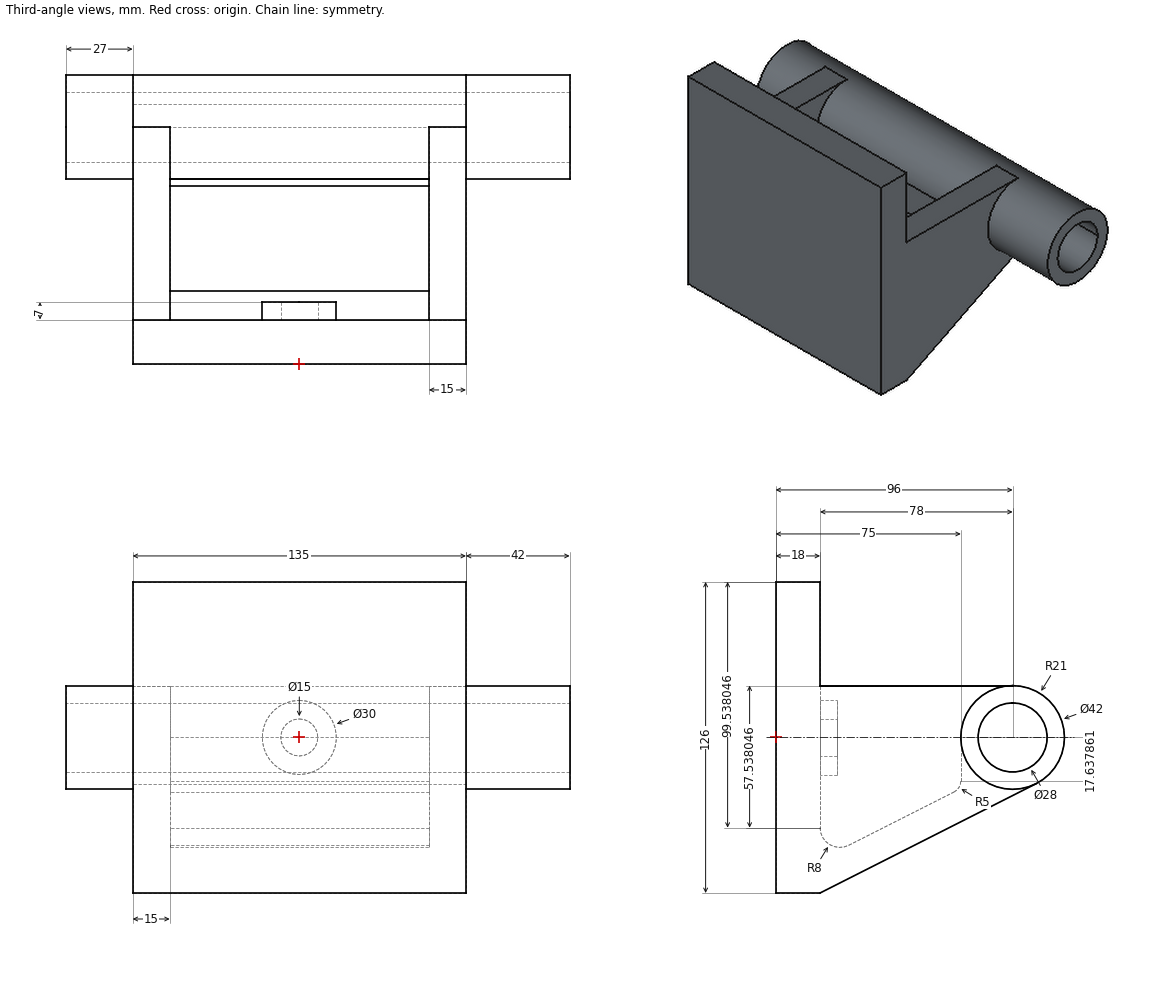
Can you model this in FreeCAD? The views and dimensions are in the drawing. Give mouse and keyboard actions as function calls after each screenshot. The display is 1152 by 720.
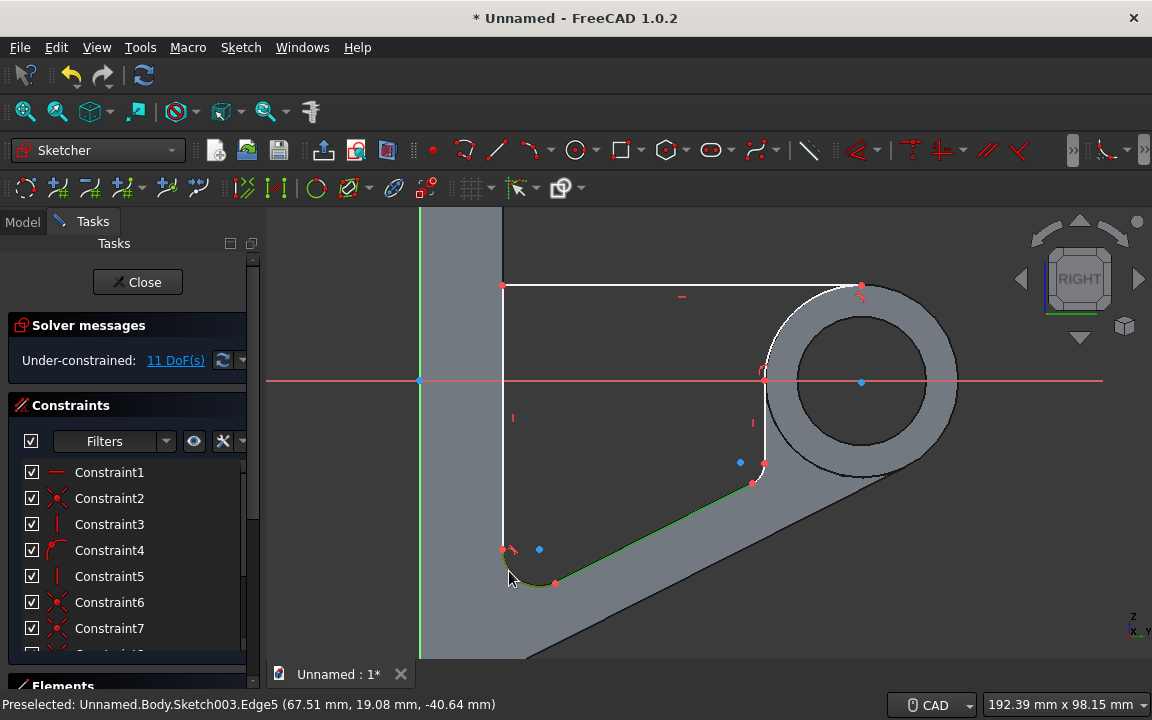
key(t)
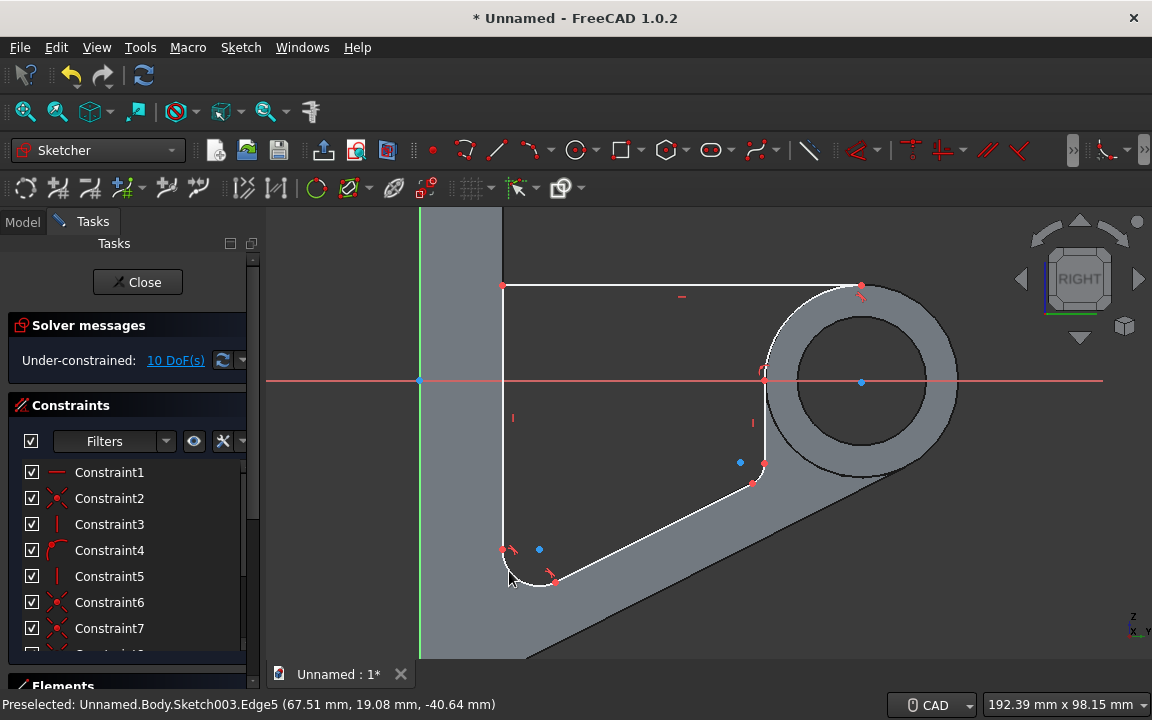
click(615, 553)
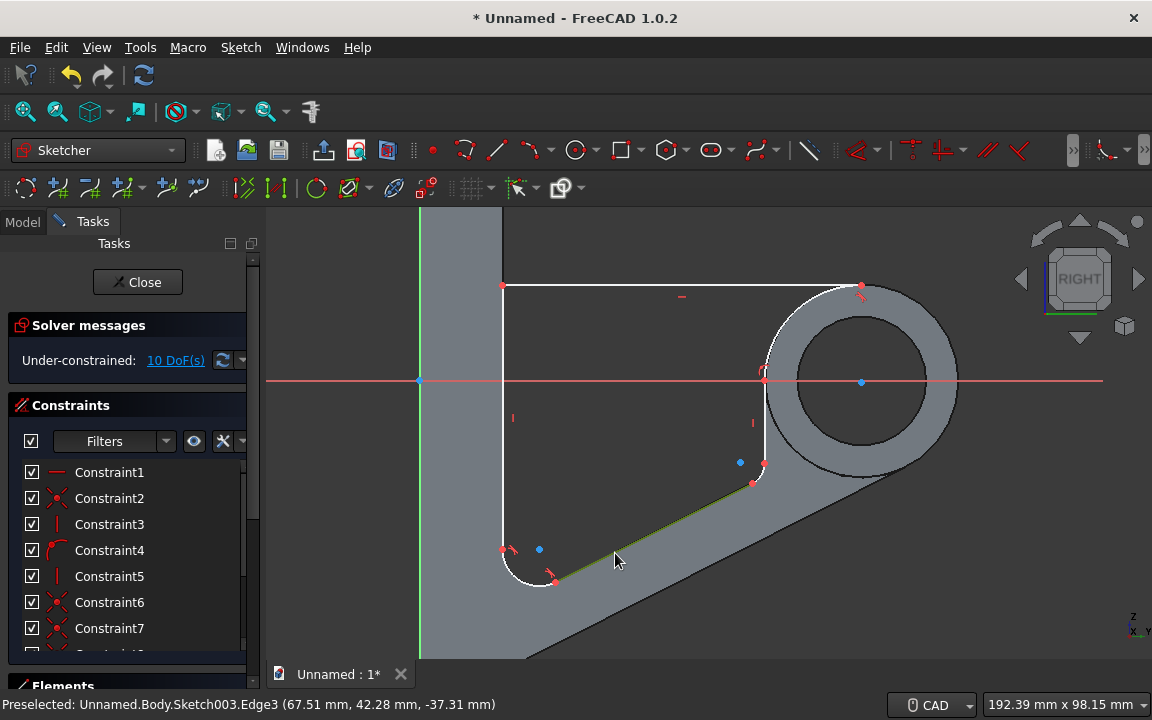
click(761, 475)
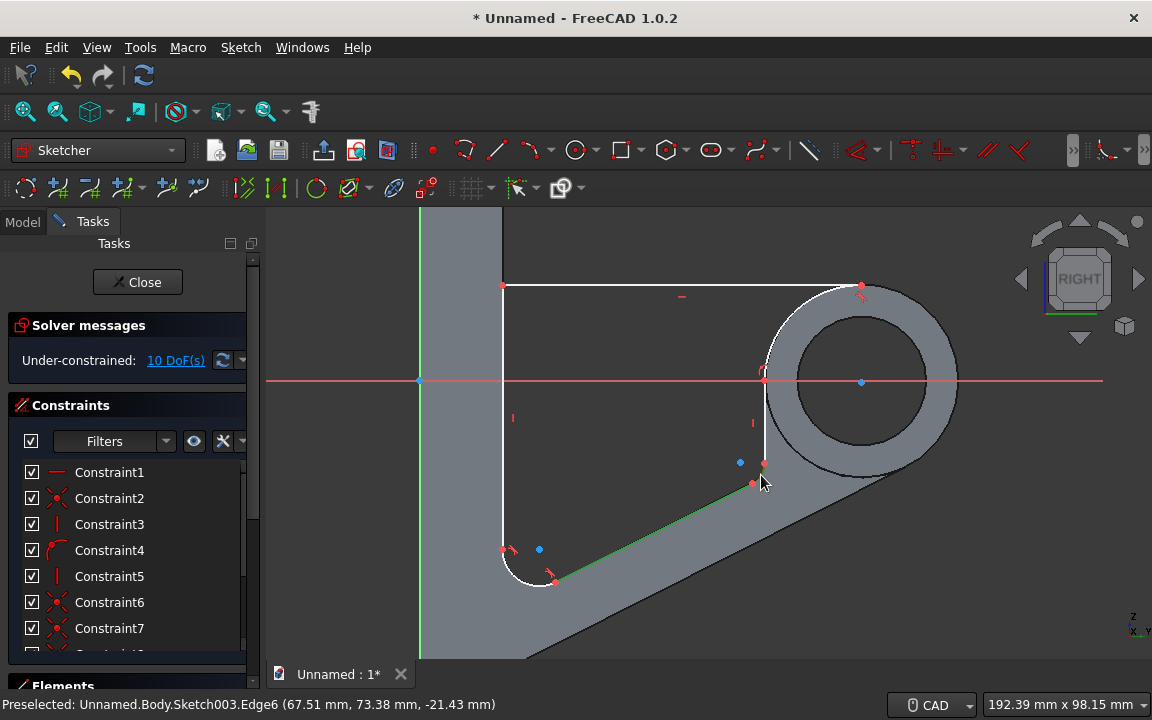
key(t)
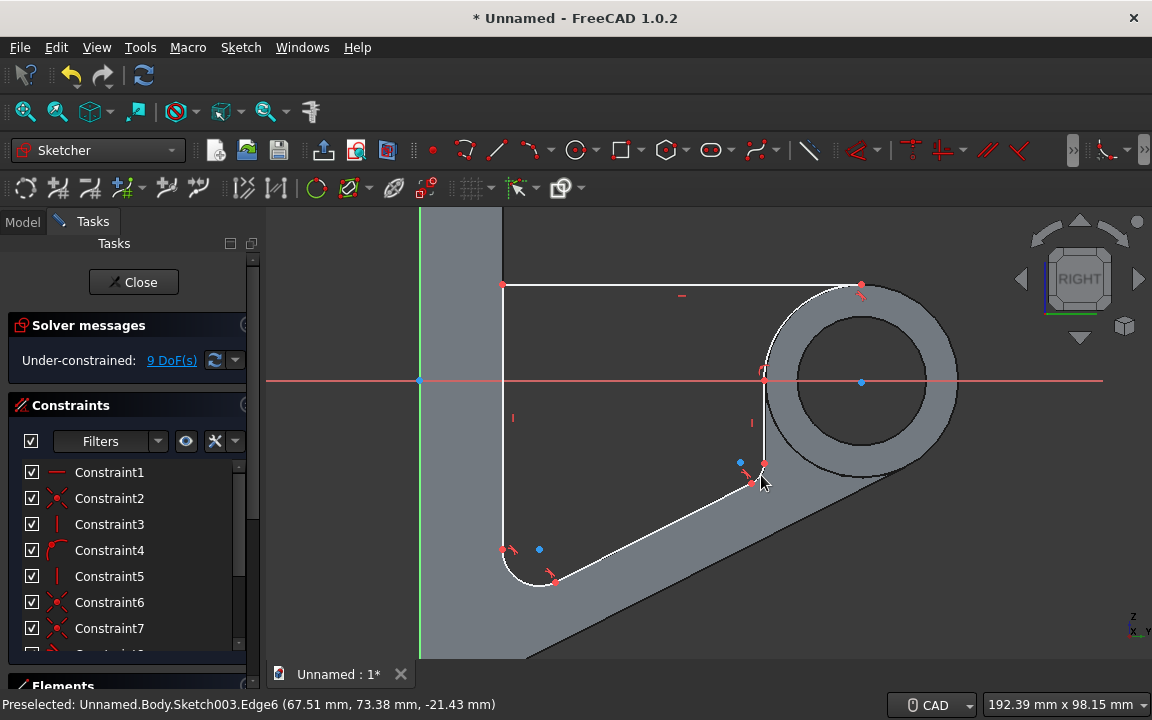
click(764, 439)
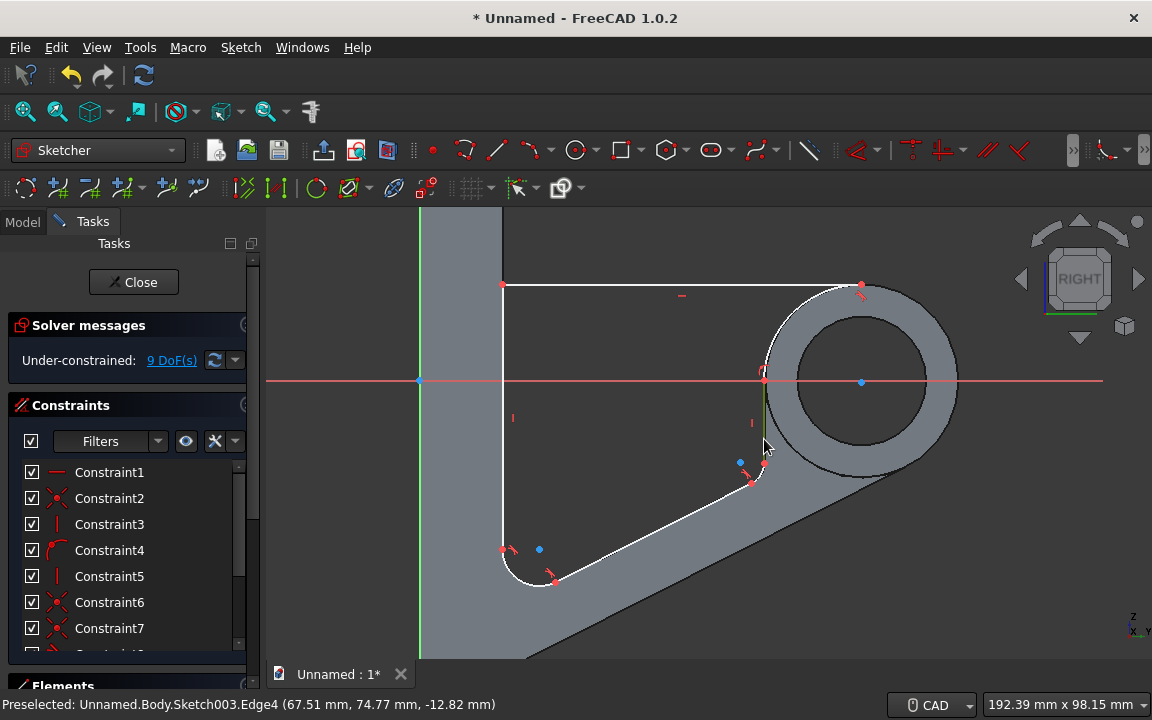
click(760, 475)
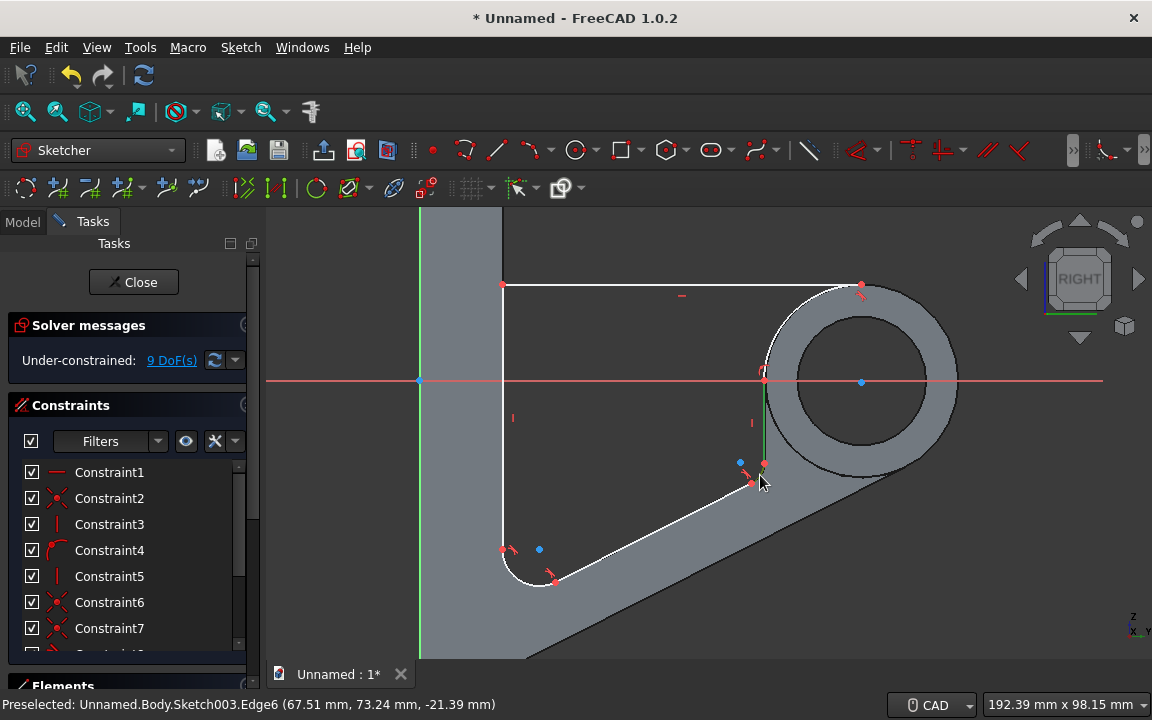
key(t)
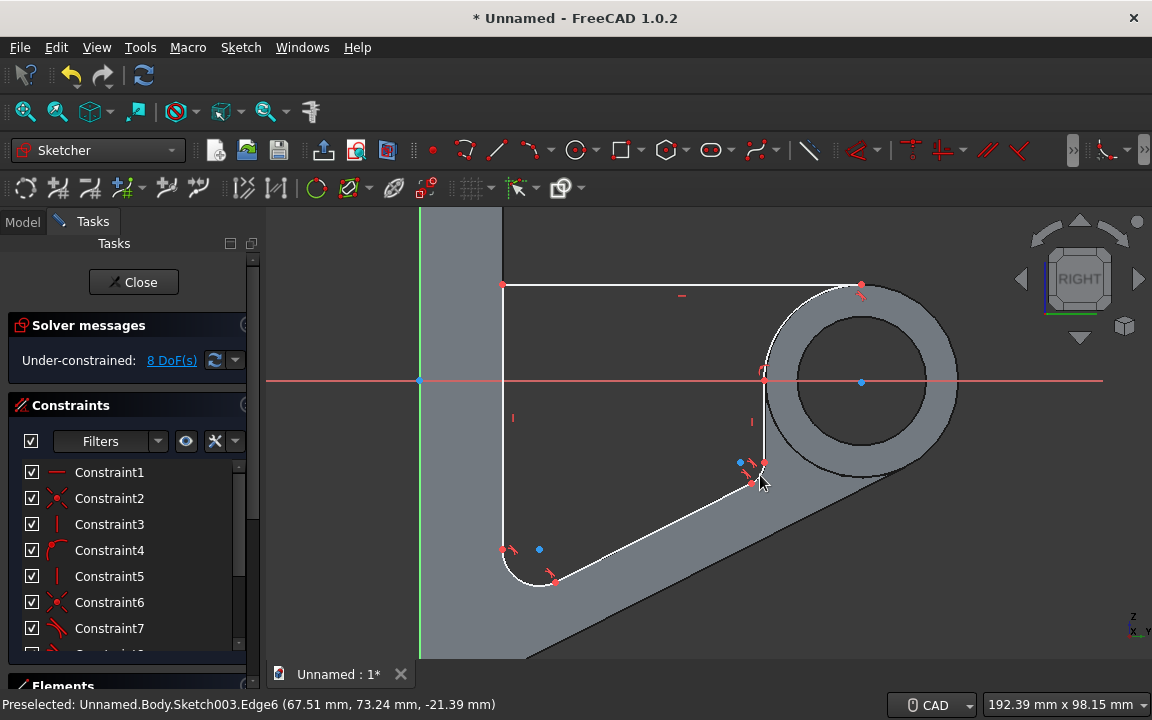
click(764, 438)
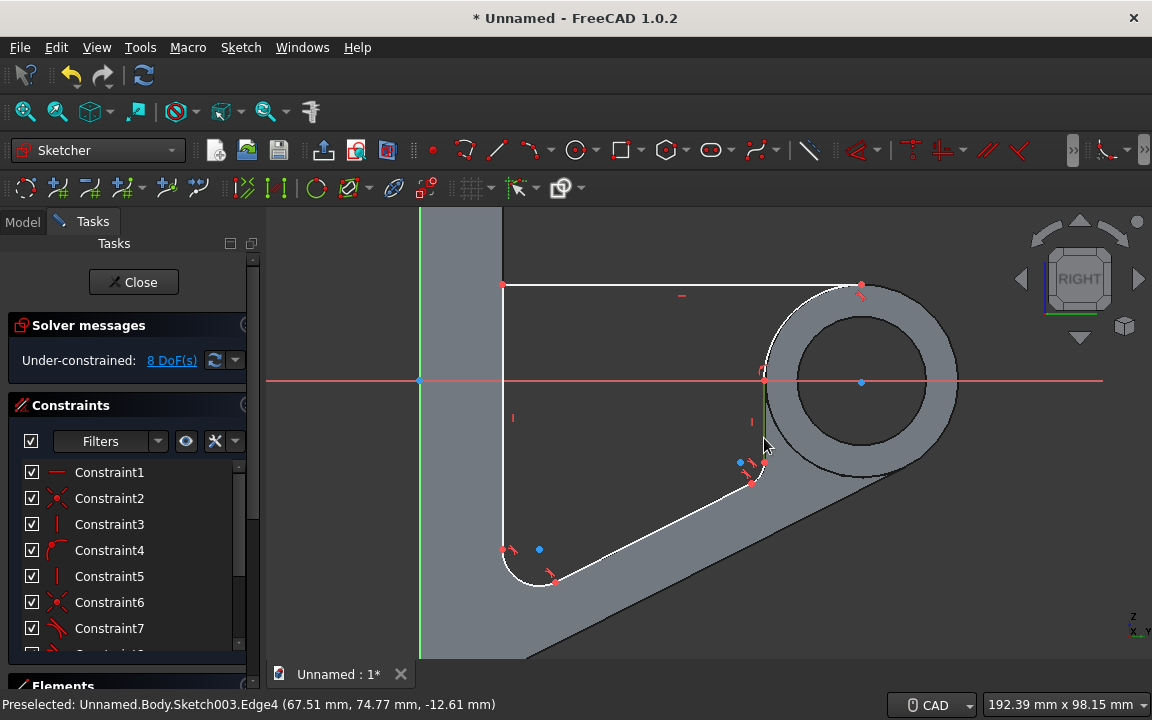
scroll(818, 295, up, 2)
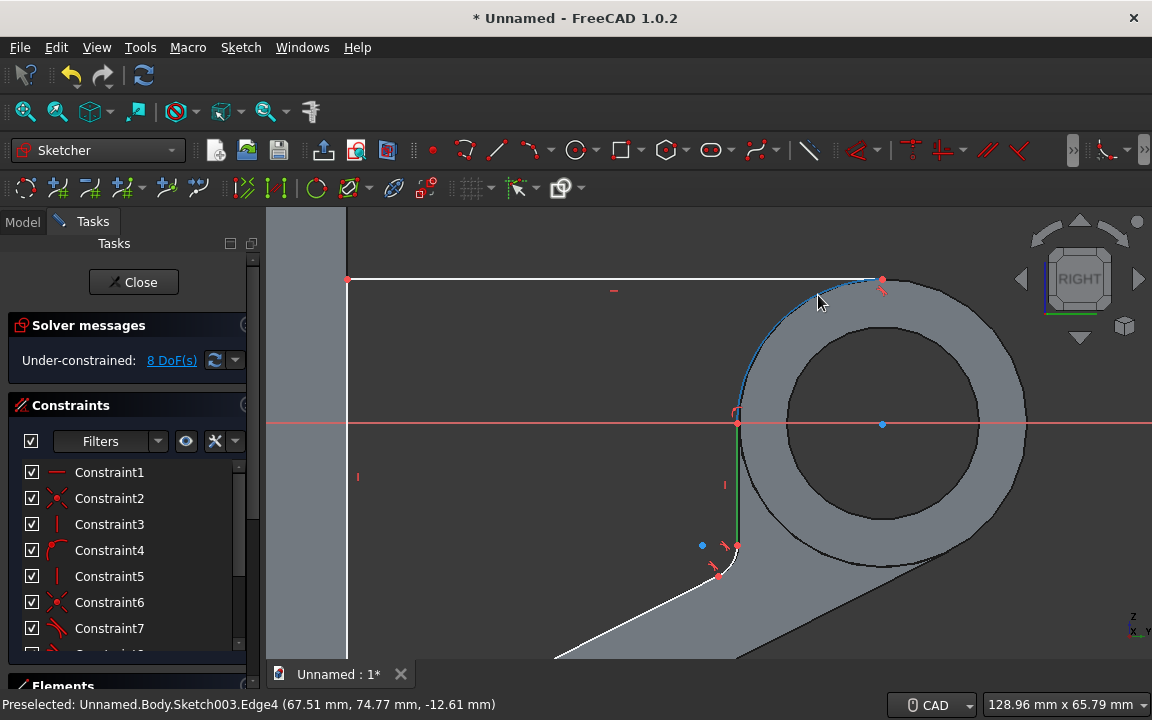
click(817, 295)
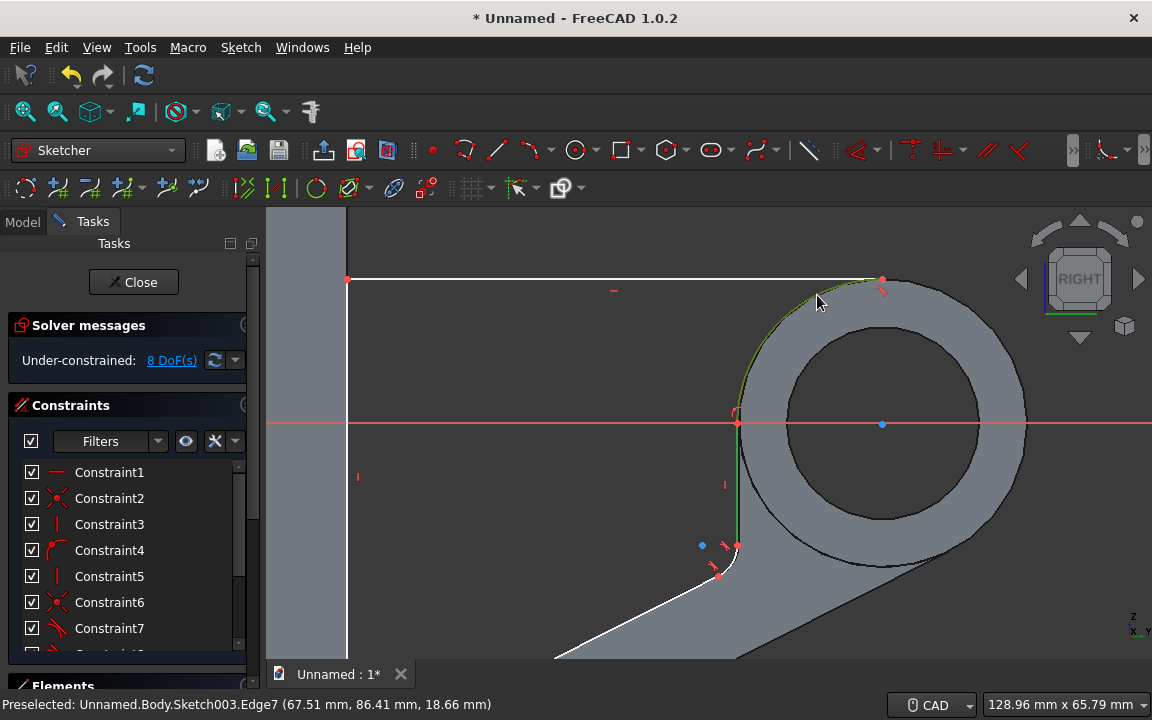
key(t)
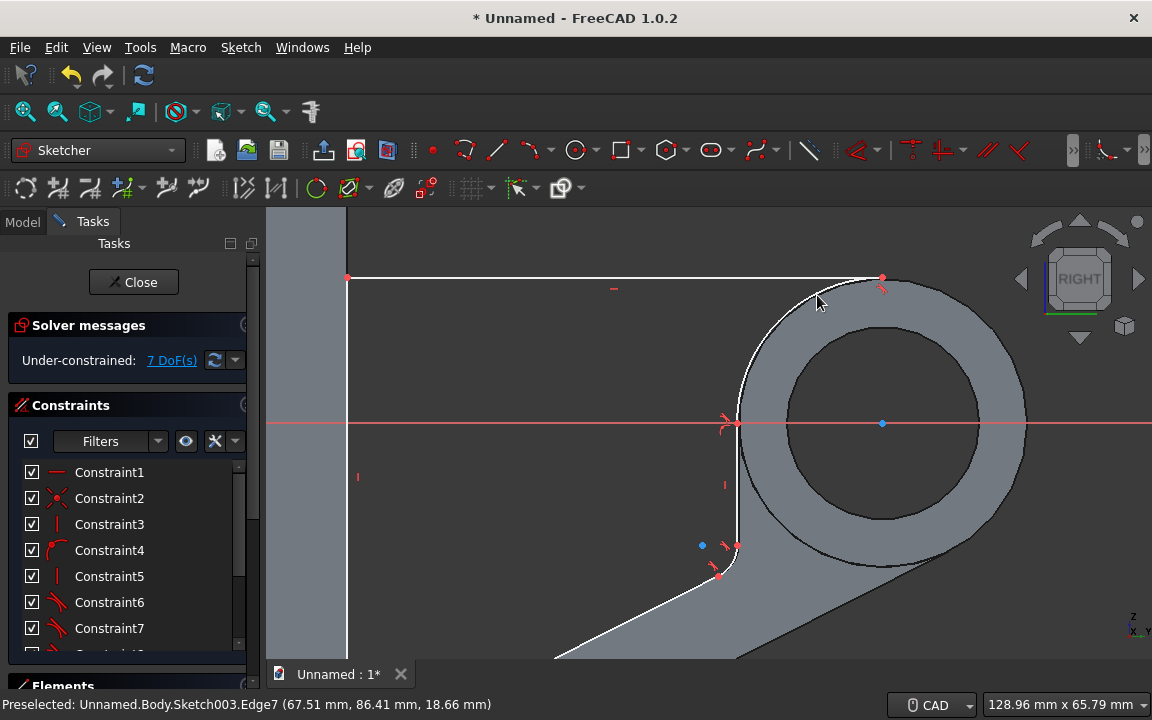
click(856, 150)